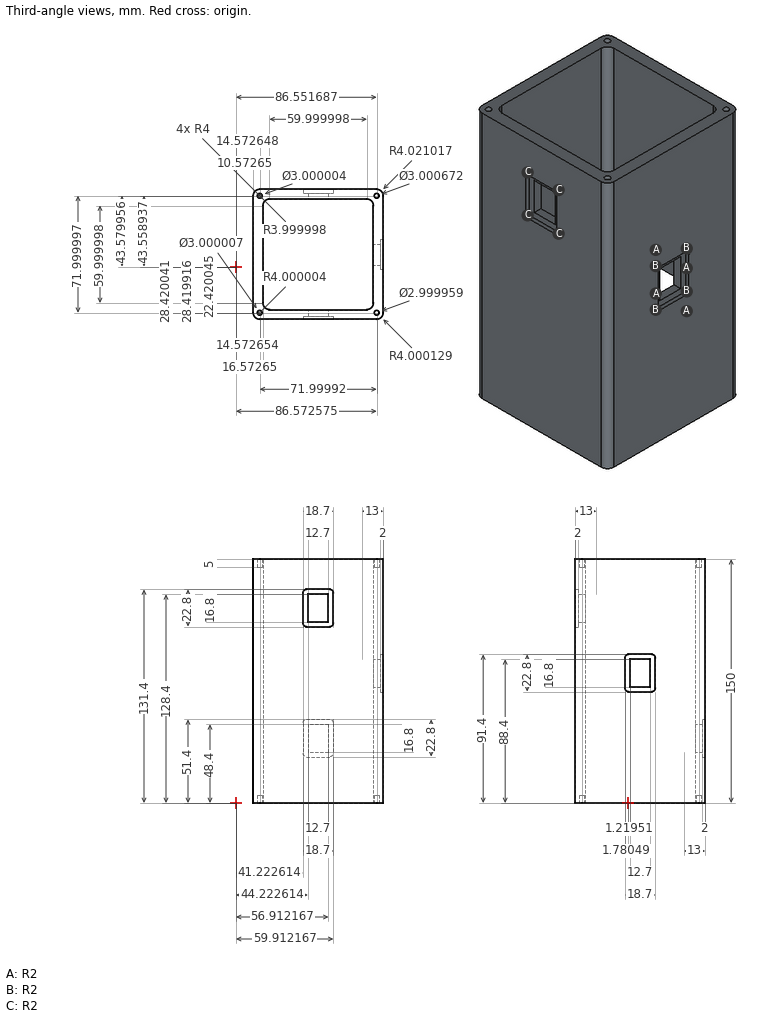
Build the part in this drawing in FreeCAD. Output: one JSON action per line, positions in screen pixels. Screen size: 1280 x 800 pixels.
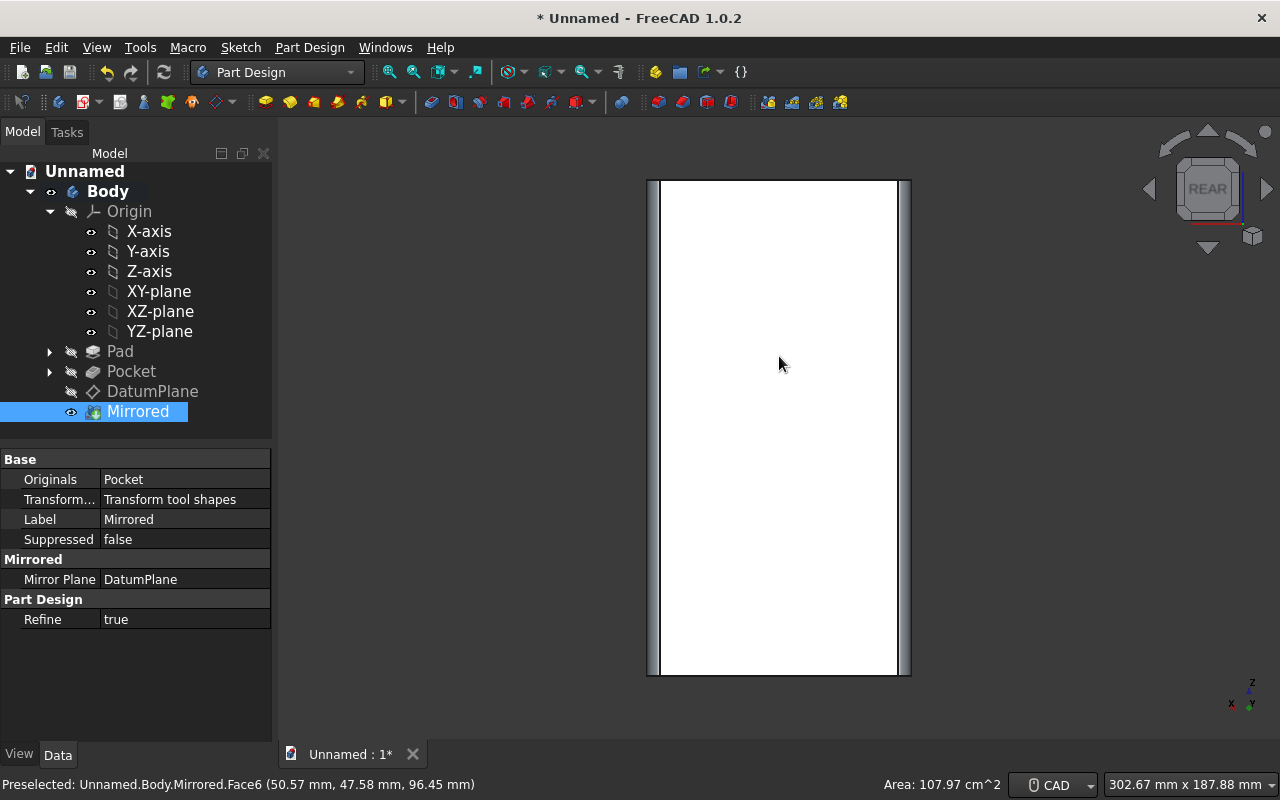
{"action": "left_click", "coordinate": [84, 102]}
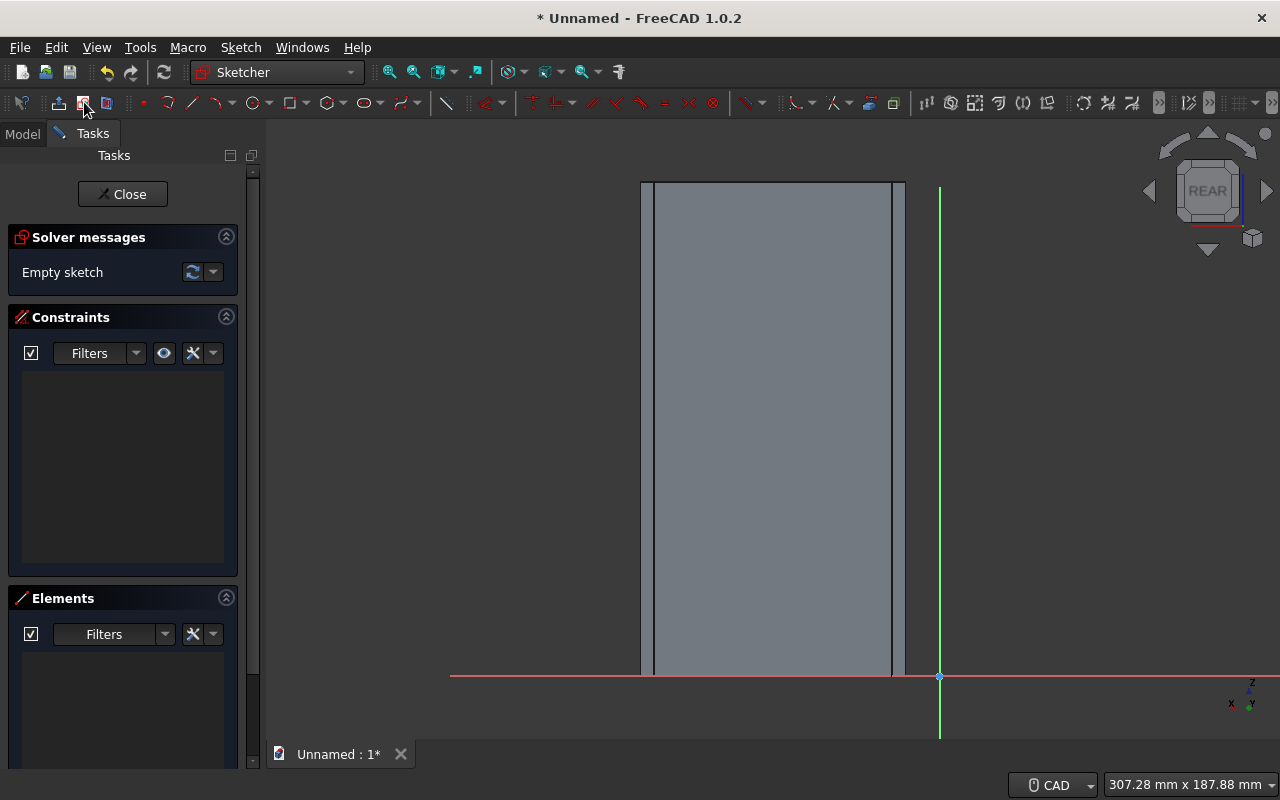
{"action": "scroll", "coordinate": [784, 563], "scroll_direction": "up", "scroll_amount": 10}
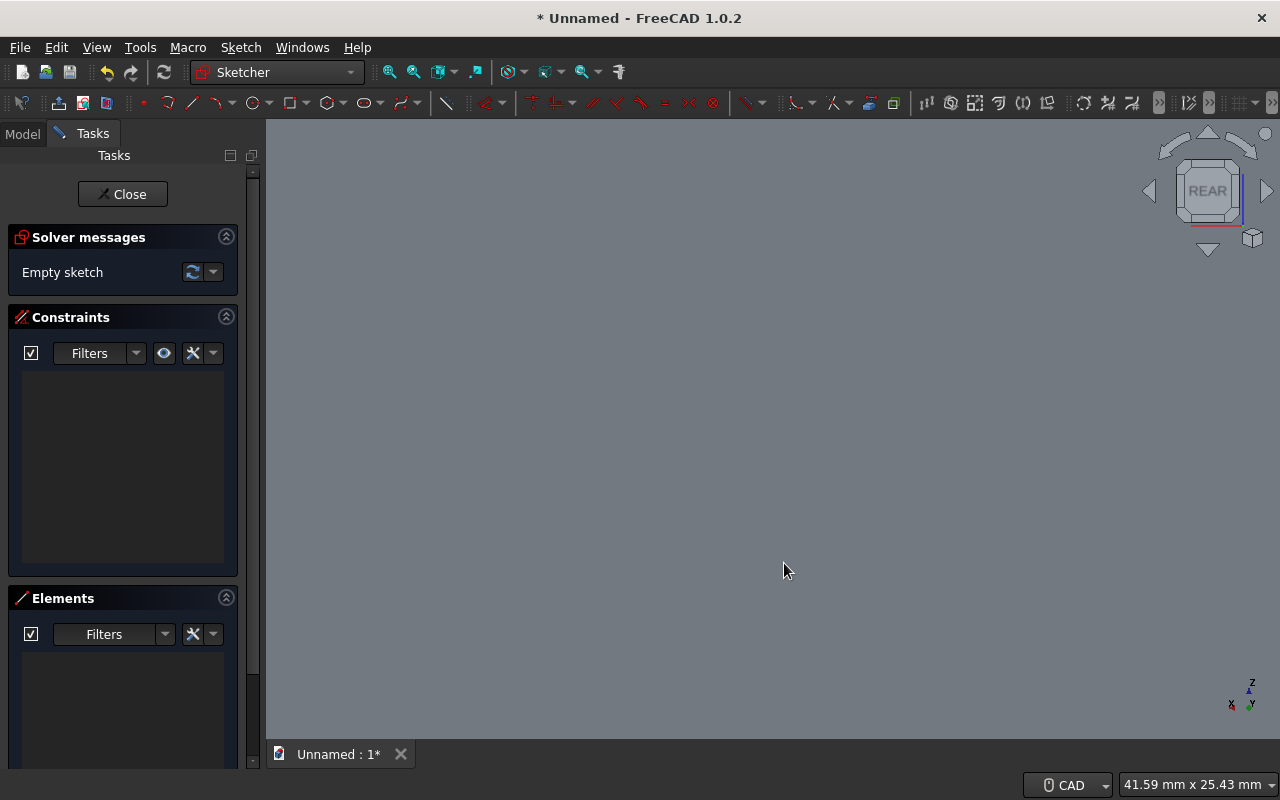
{"action": "left_click", "coordinate": [290, 104]}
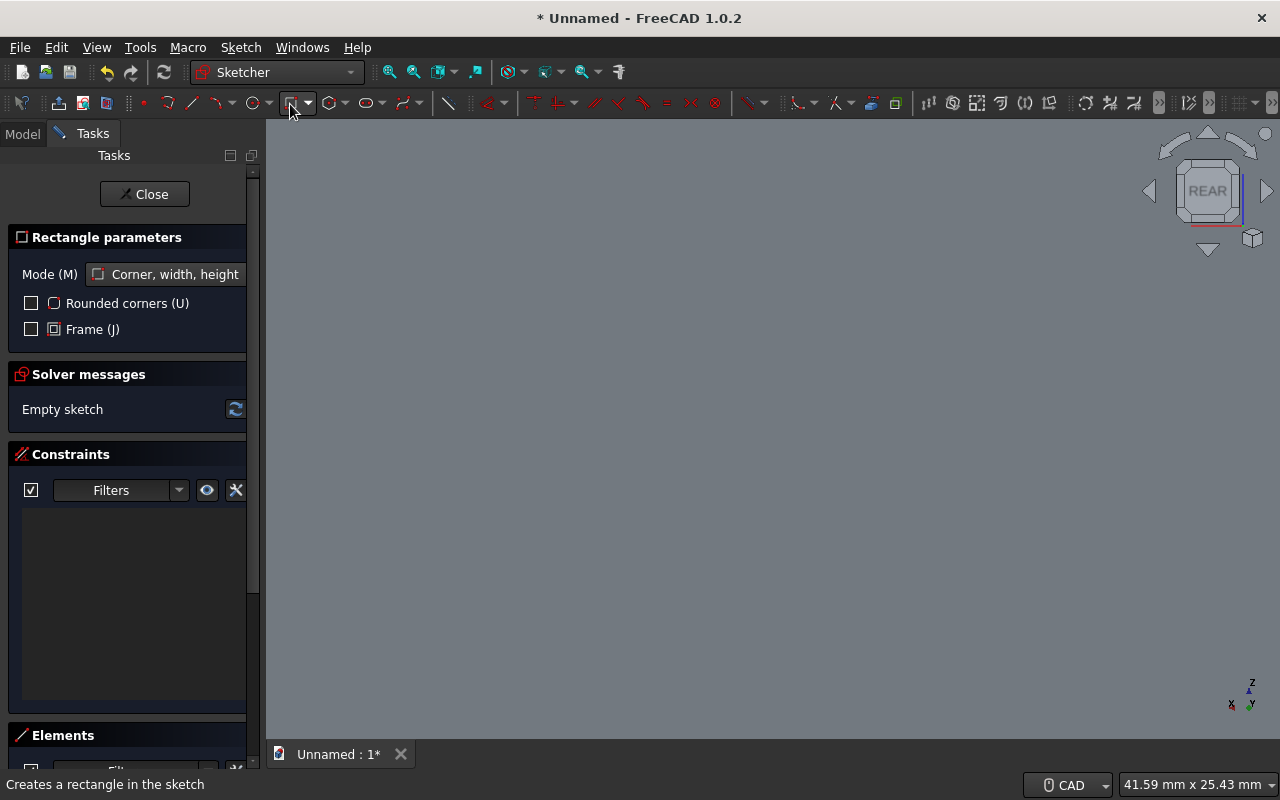
{"action": "left_click", "coordinate": [545, 217]}
{"action": "left_click", "coordinate": [855, 627]}
{"action": "key", "text": "Escape"}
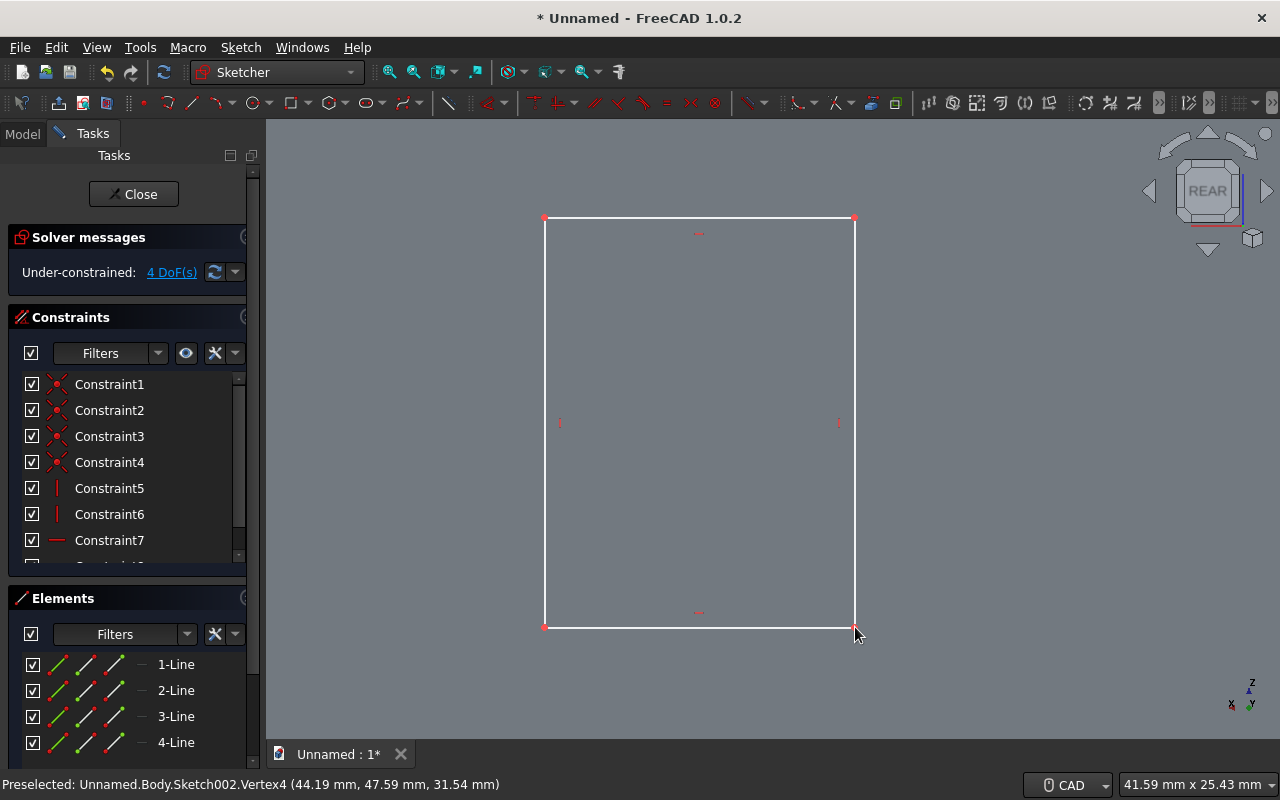
{"action": "left_click", "coordinate": [488, 104]}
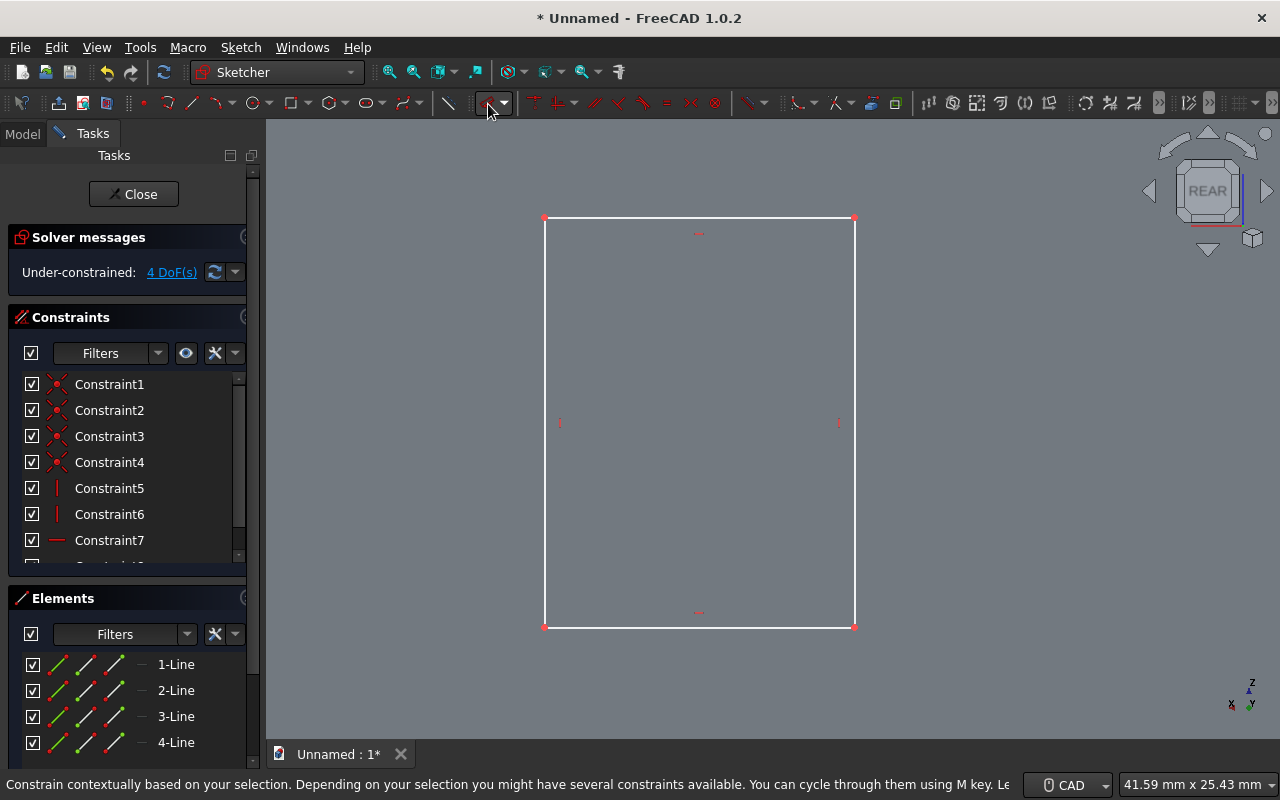
{"action": "left_click", "coordinate": [545, 341]}
{"action": "left_click", "coordinate": [511, 423]}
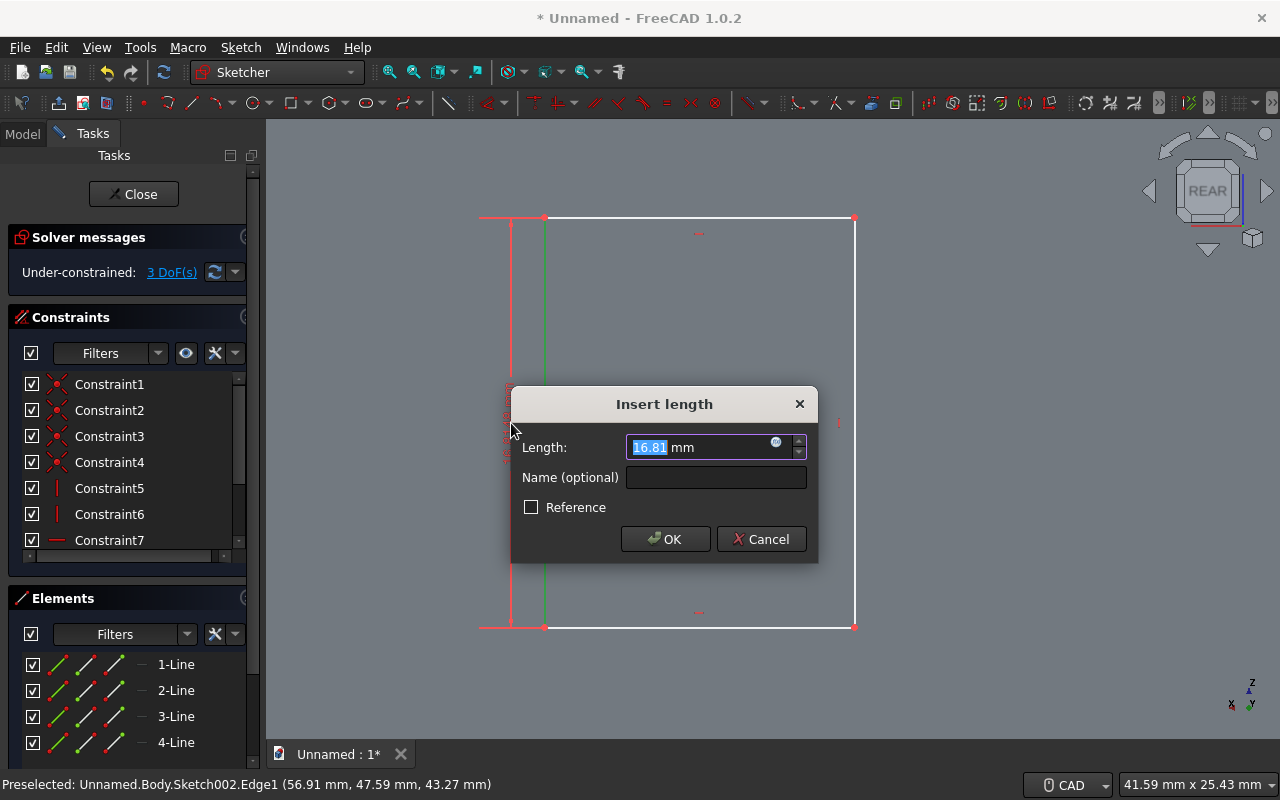
{"action": "type", "text": "16.8"}
{"action": "key", "text": "Return"}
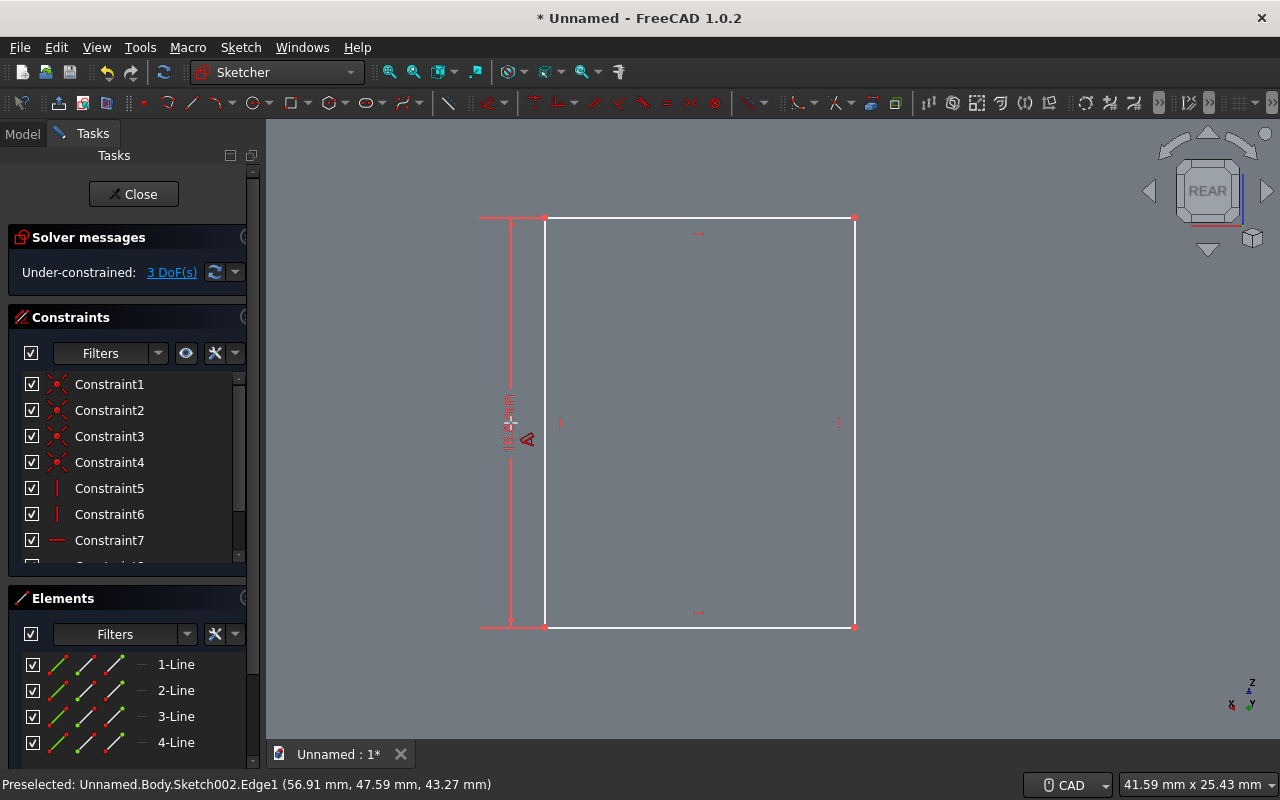
{"action": "left_click", "coordinate": [638, 628]}
{"action": "left_click", "coordinate": [700, 662]}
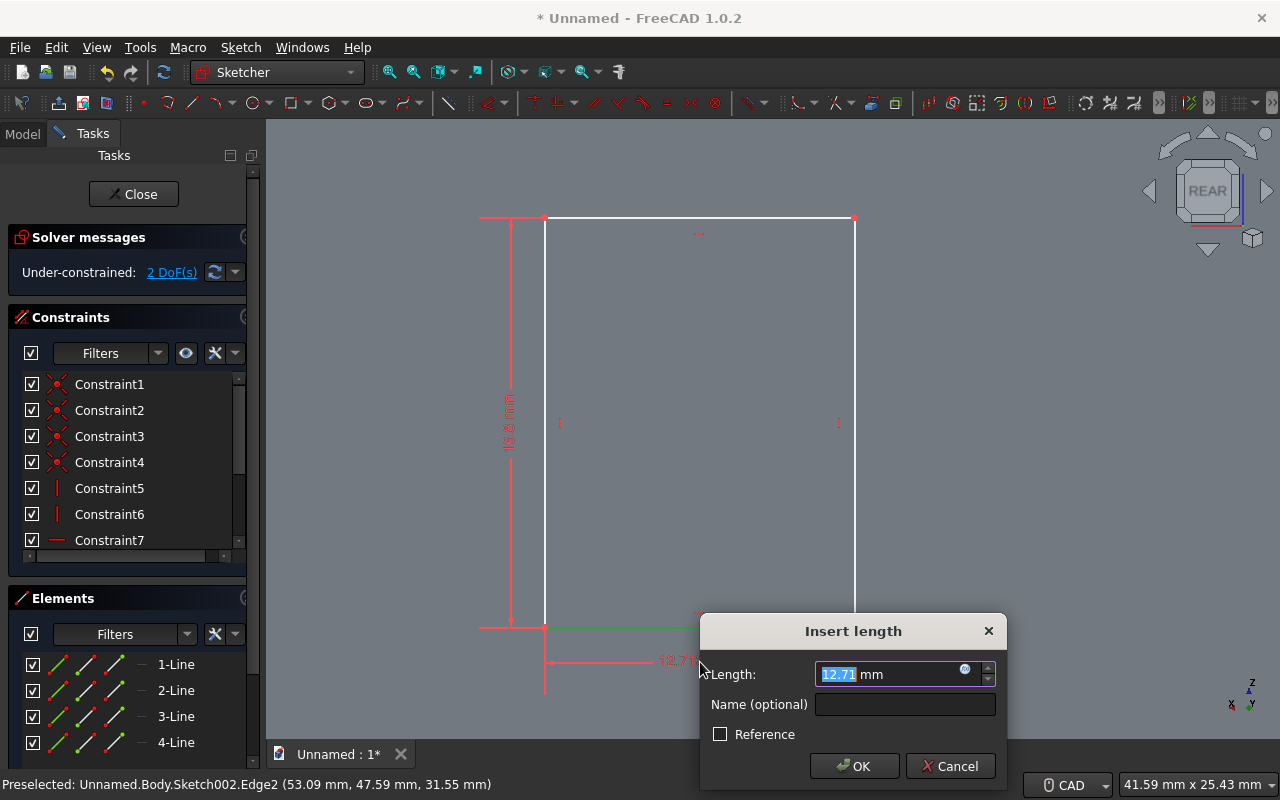
{"action": "type", "text": "12.7"}
{"action": "key", "text": "Return"}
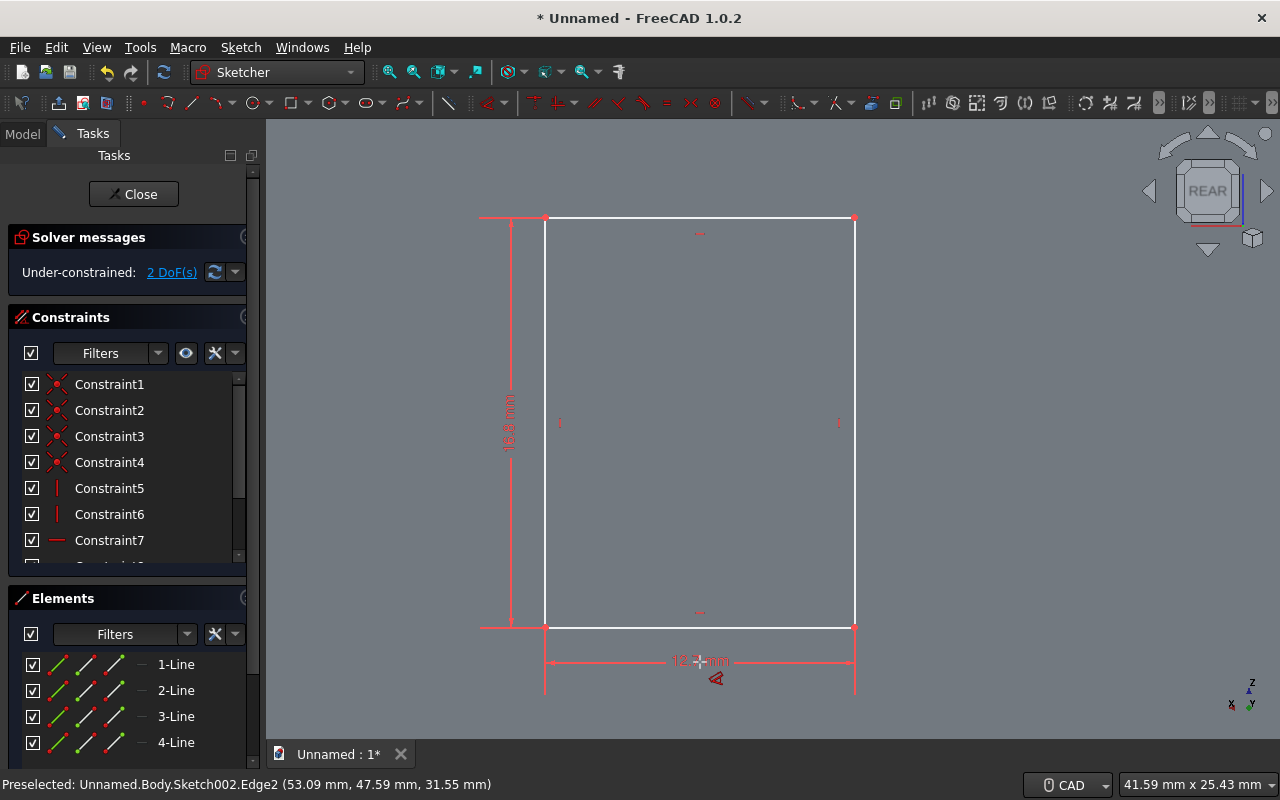
{"action": "left_click", "coordinate": [545, 218]}
{"action": "left_click", "coordinate": [511, 465]}